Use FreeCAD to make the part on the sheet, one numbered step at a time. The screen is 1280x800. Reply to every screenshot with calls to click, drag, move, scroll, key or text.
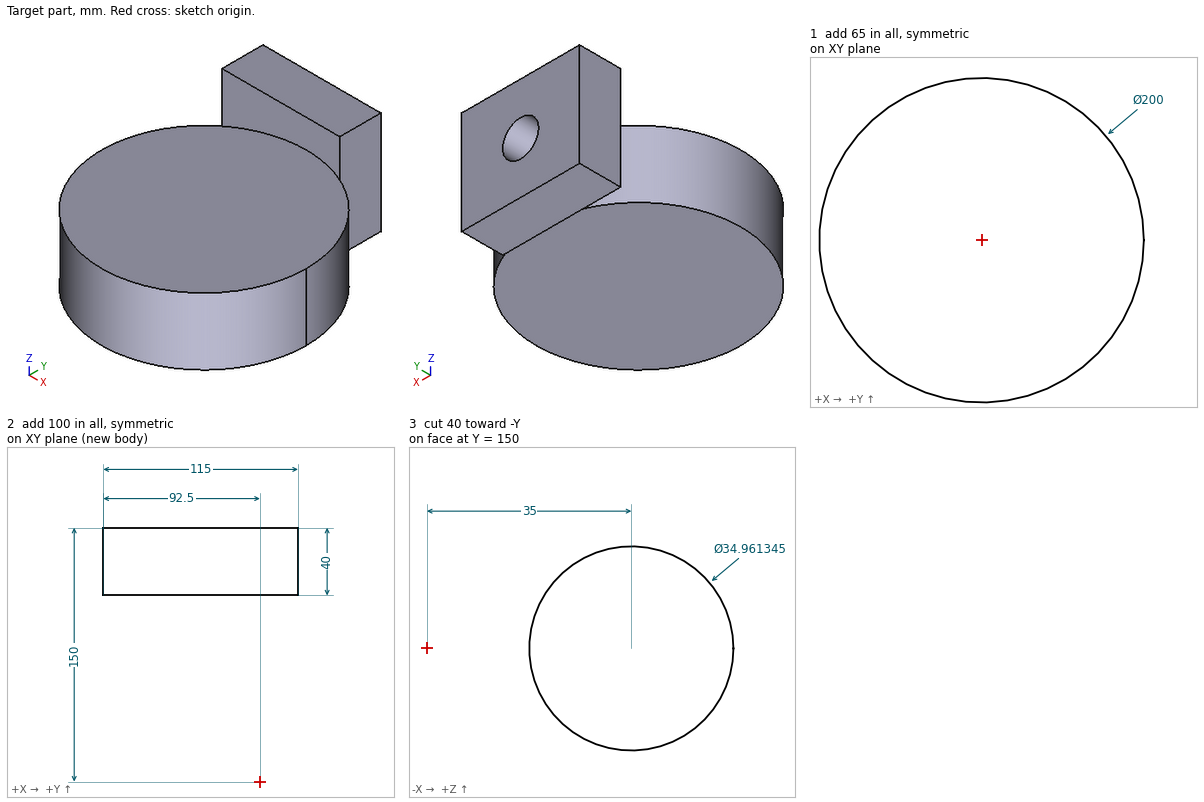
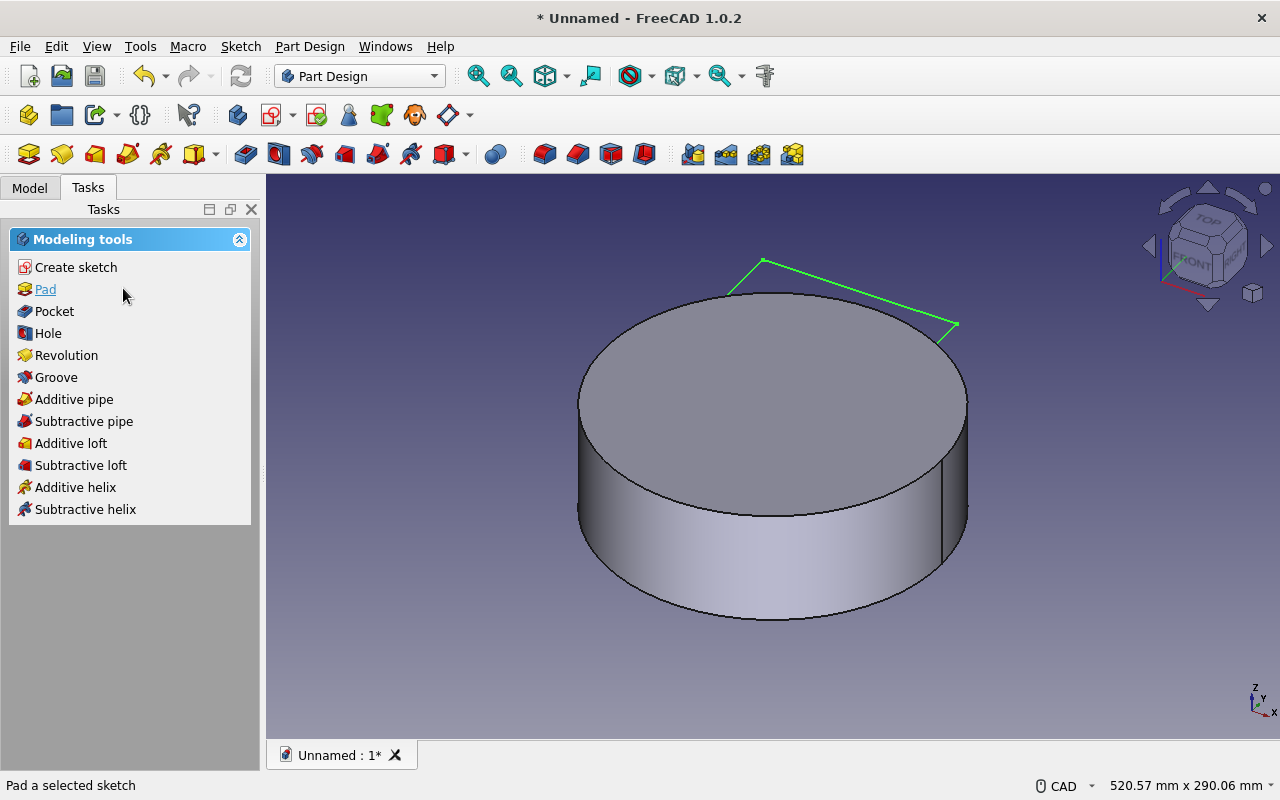
click(29, 154)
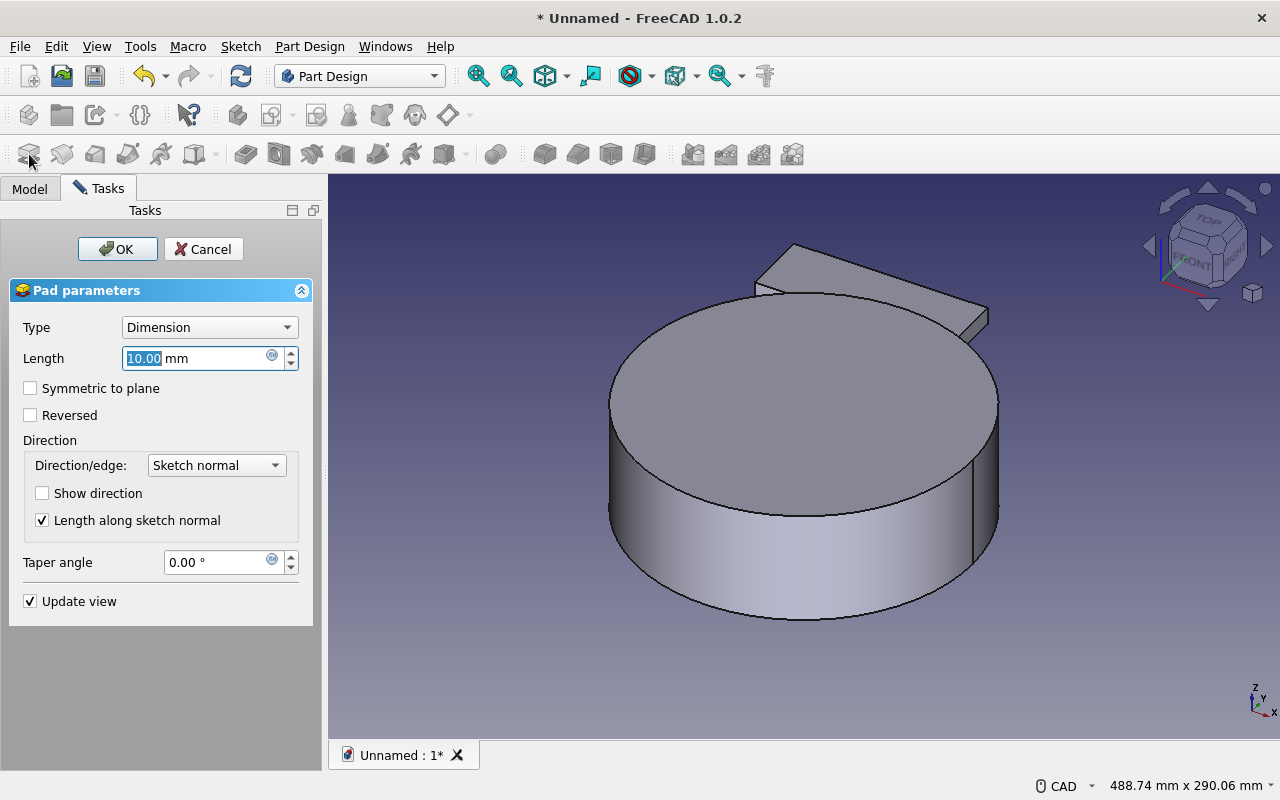
text(100)
key(Tab)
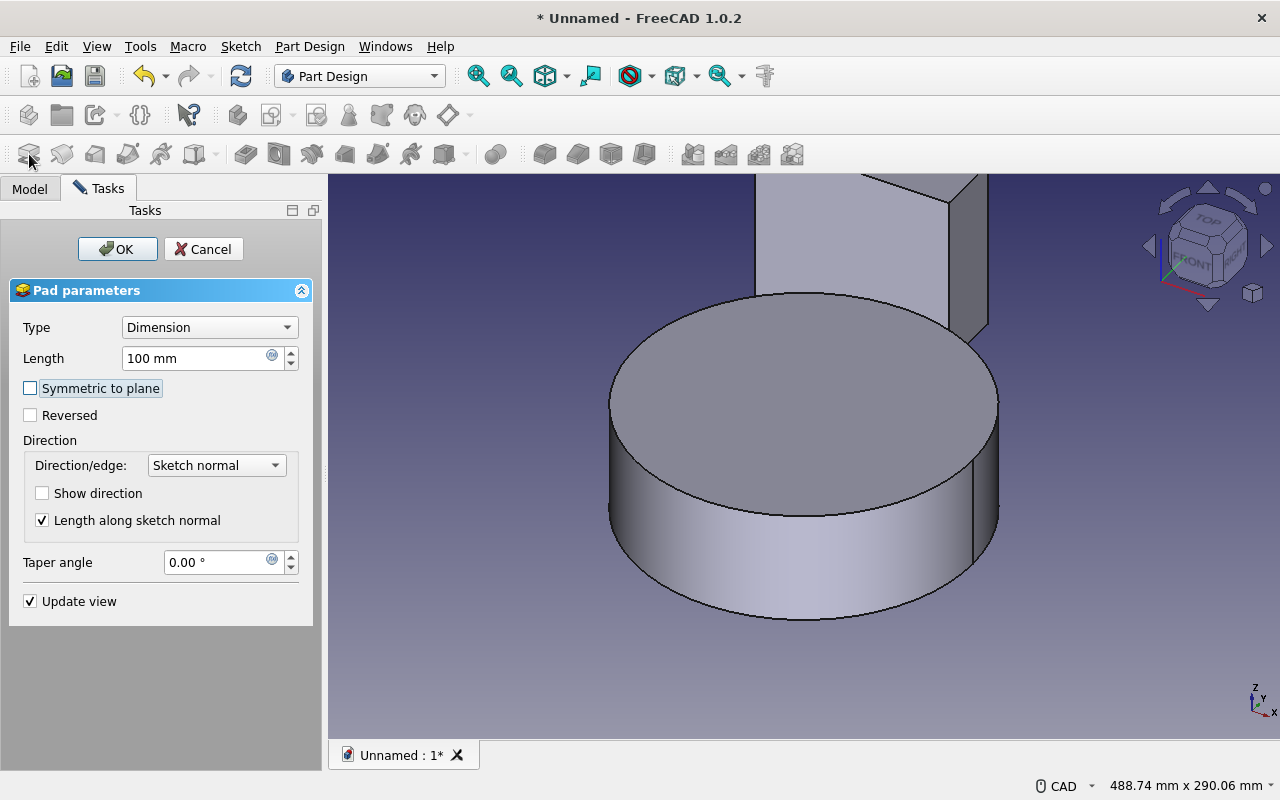
click(31, 388)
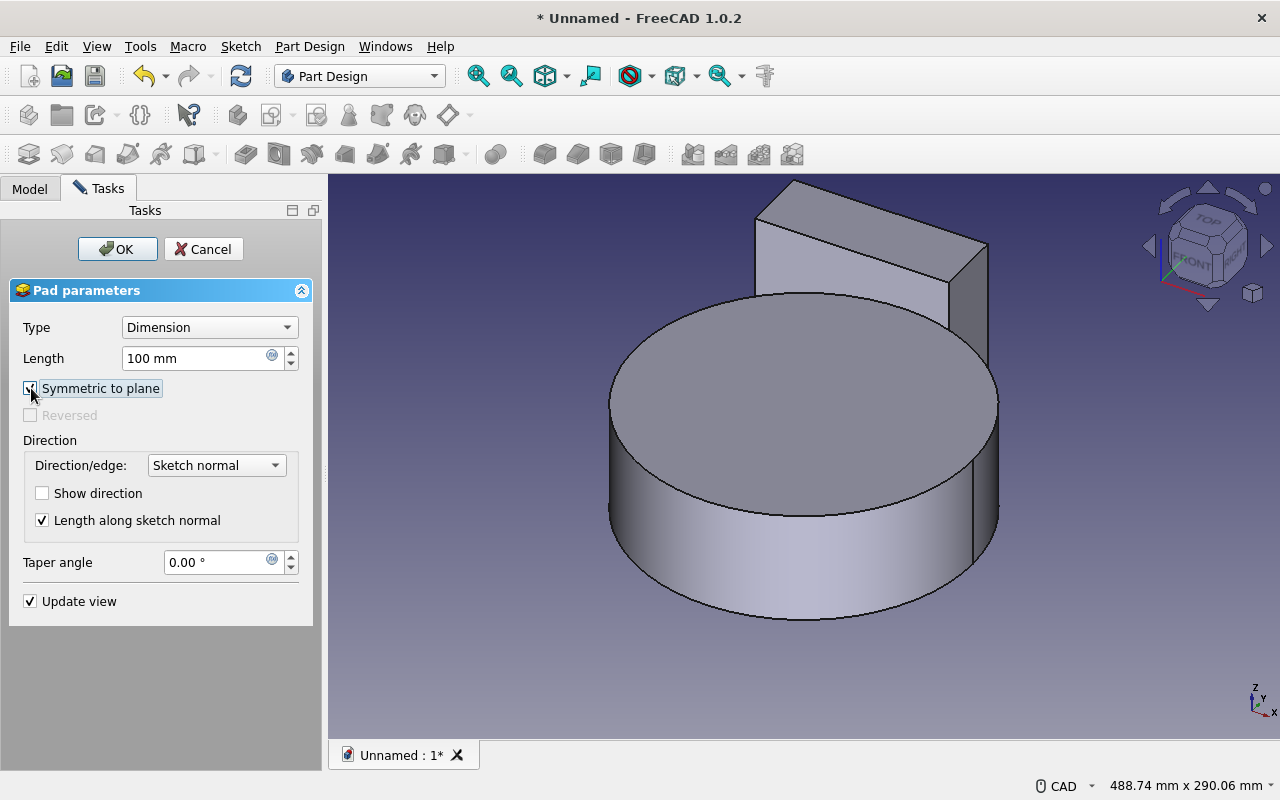
click(118, 249)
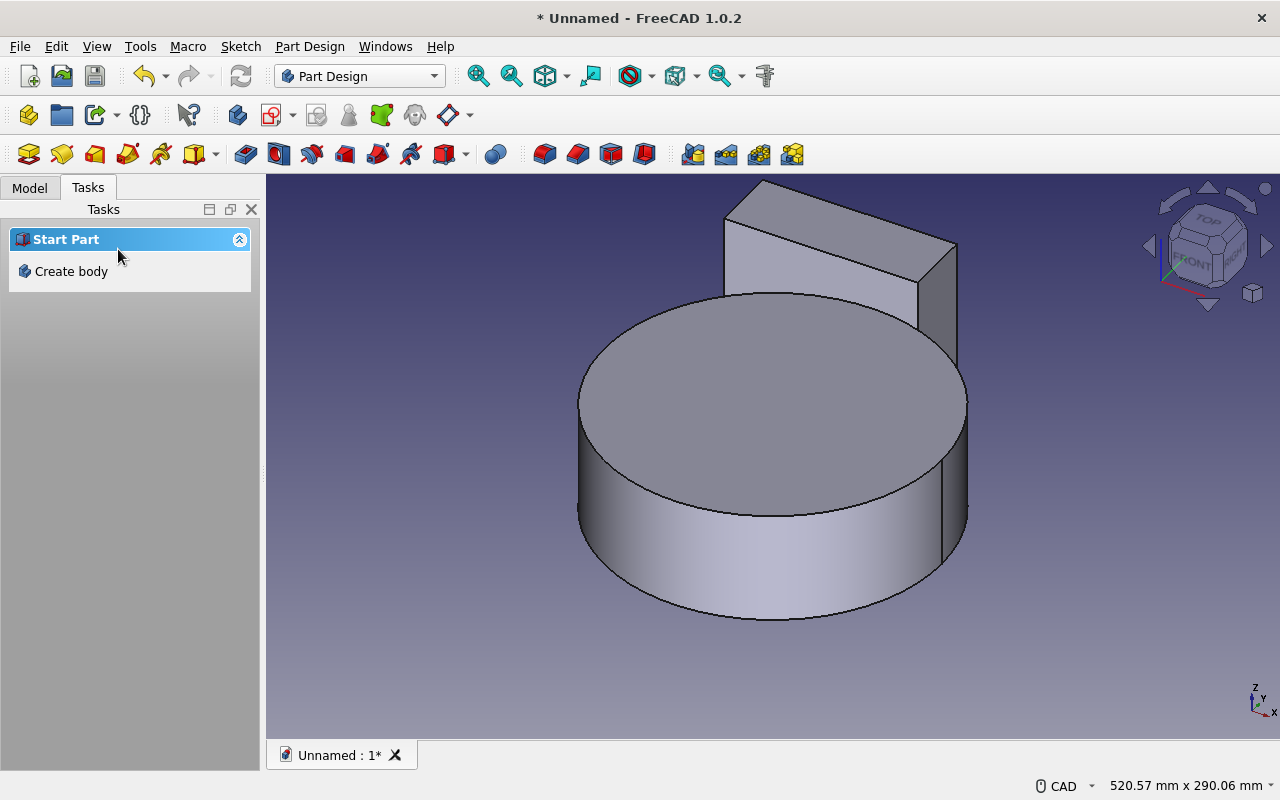
key(4)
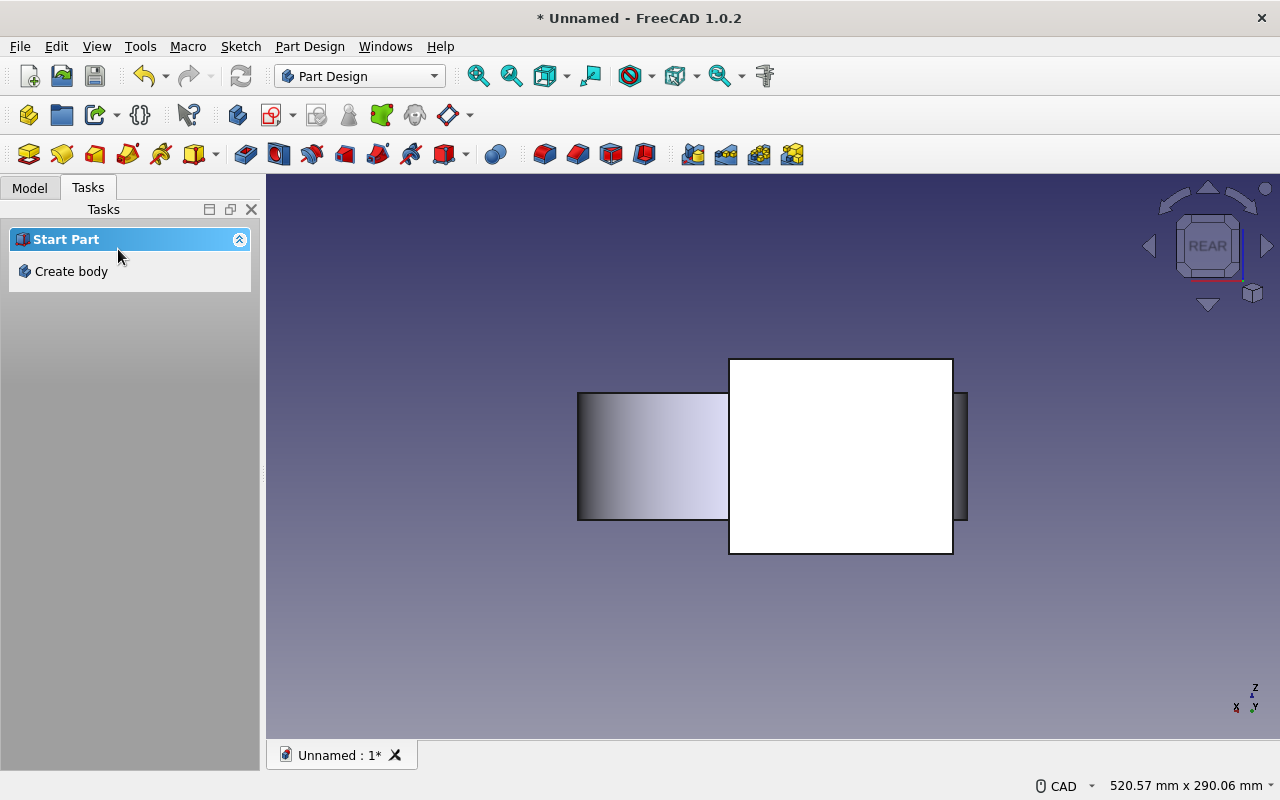
click(479, 76)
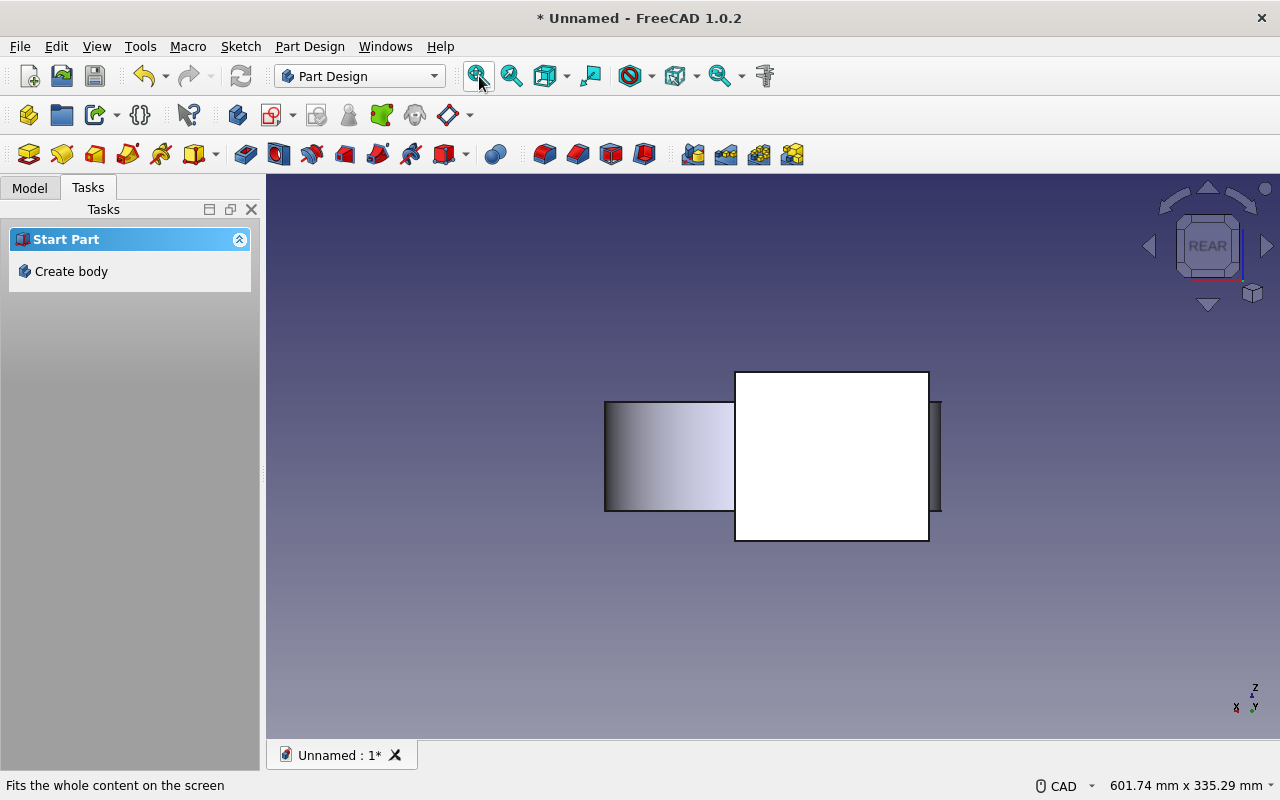
click(832, 456)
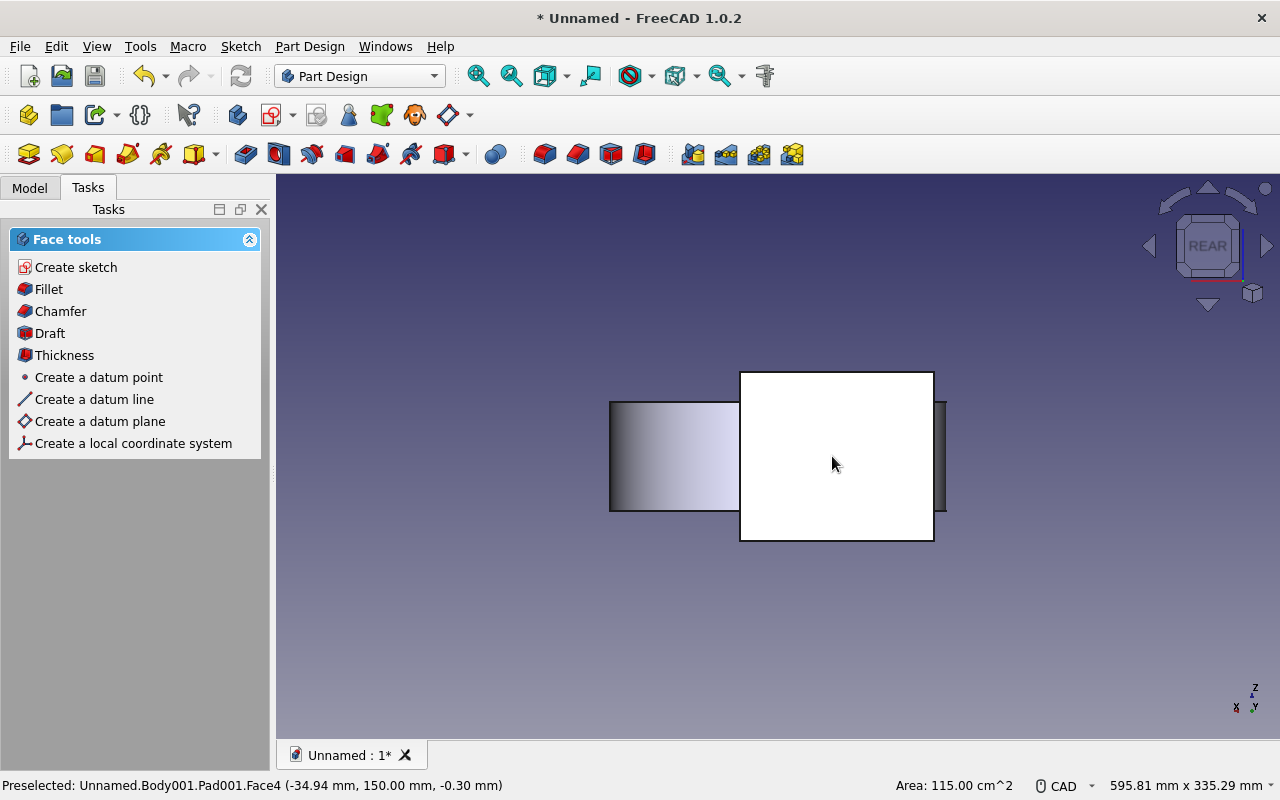
click(270, 116)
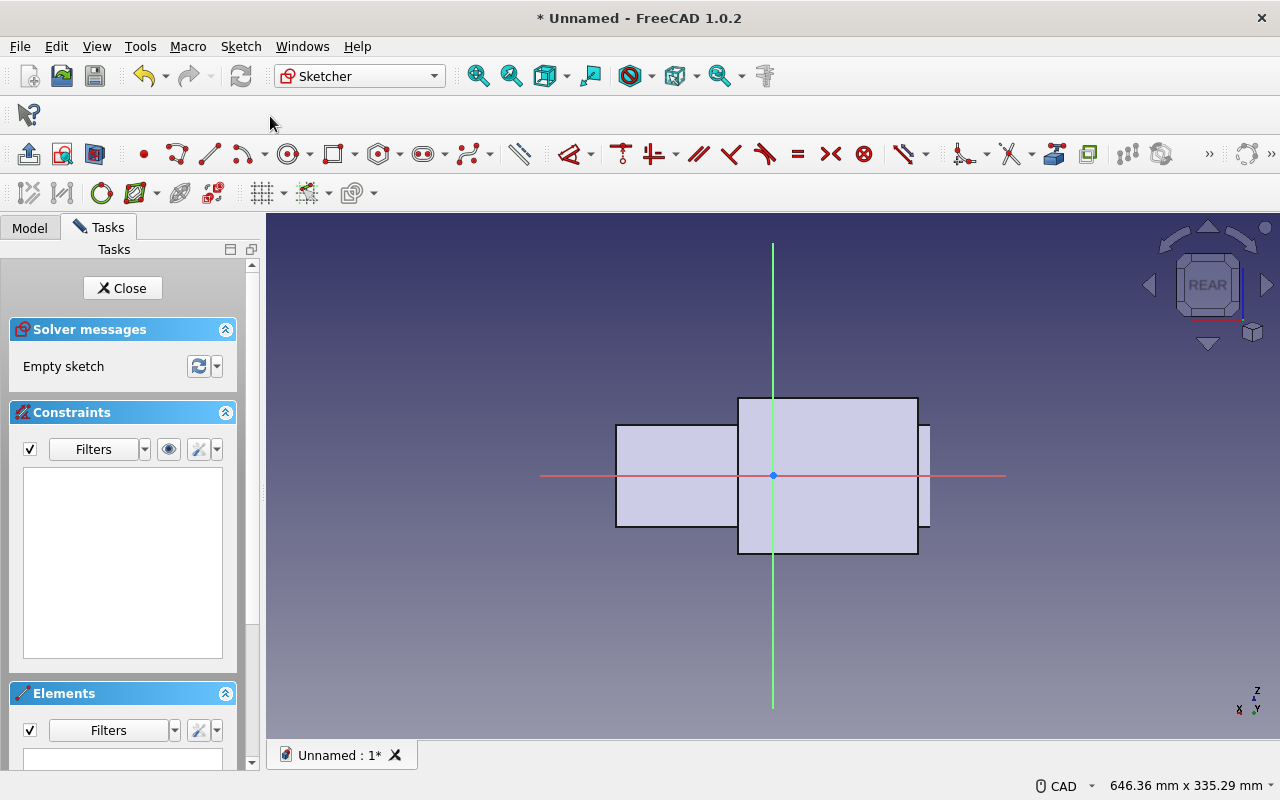
scroll(836, 476, up, 9)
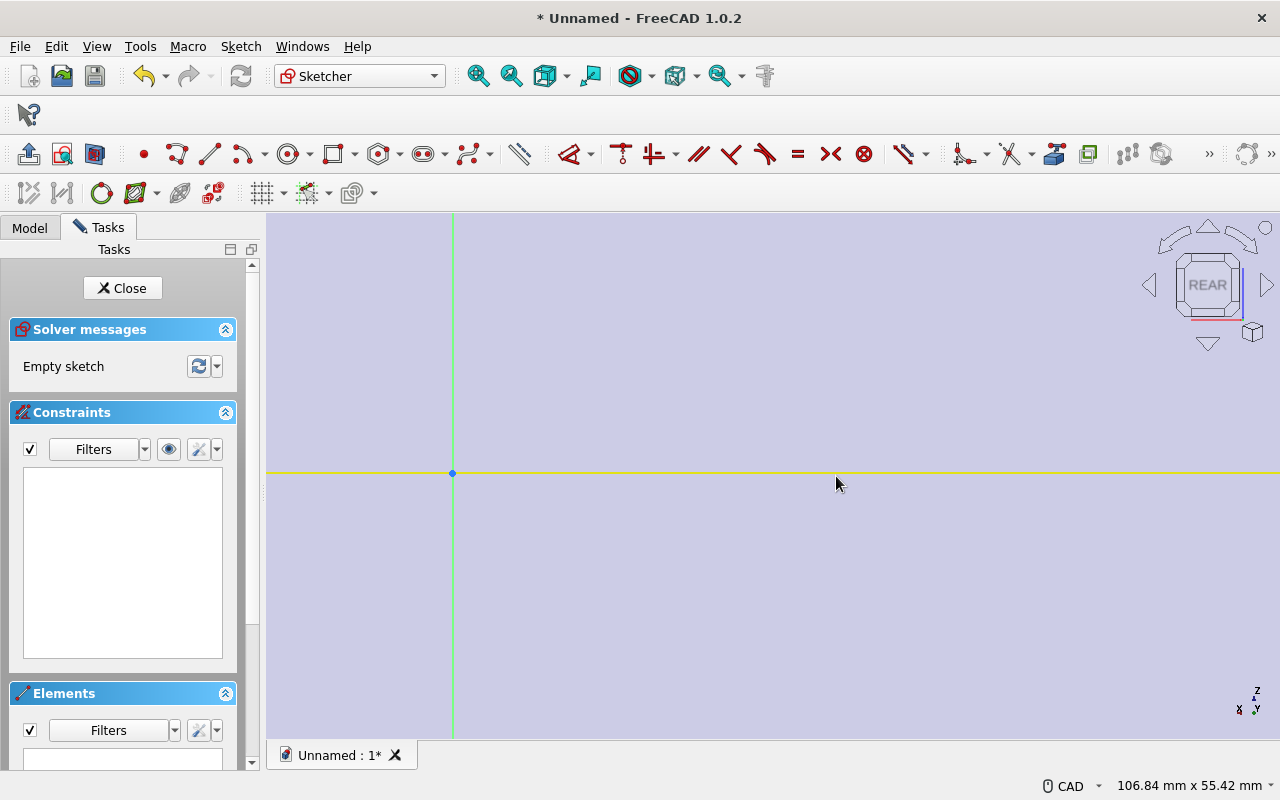
key(g)
key(c)